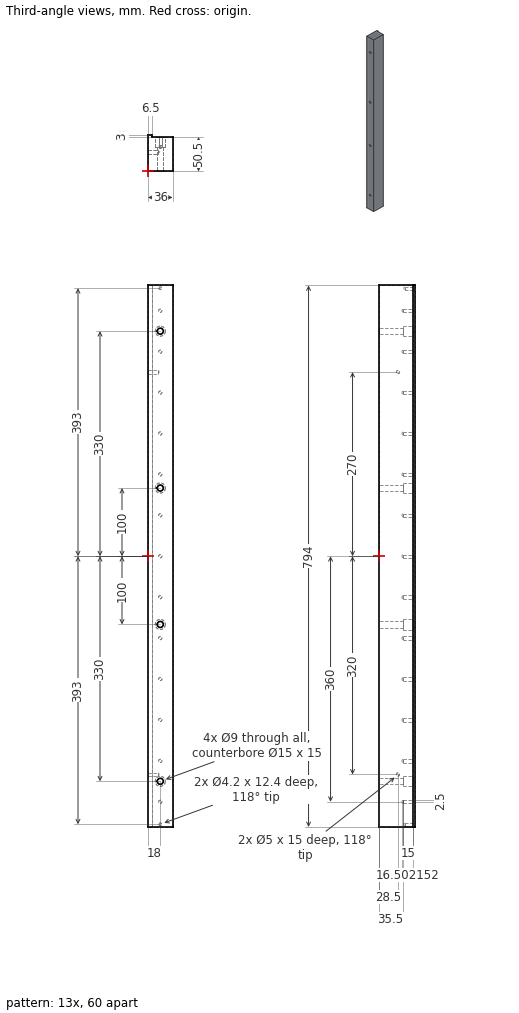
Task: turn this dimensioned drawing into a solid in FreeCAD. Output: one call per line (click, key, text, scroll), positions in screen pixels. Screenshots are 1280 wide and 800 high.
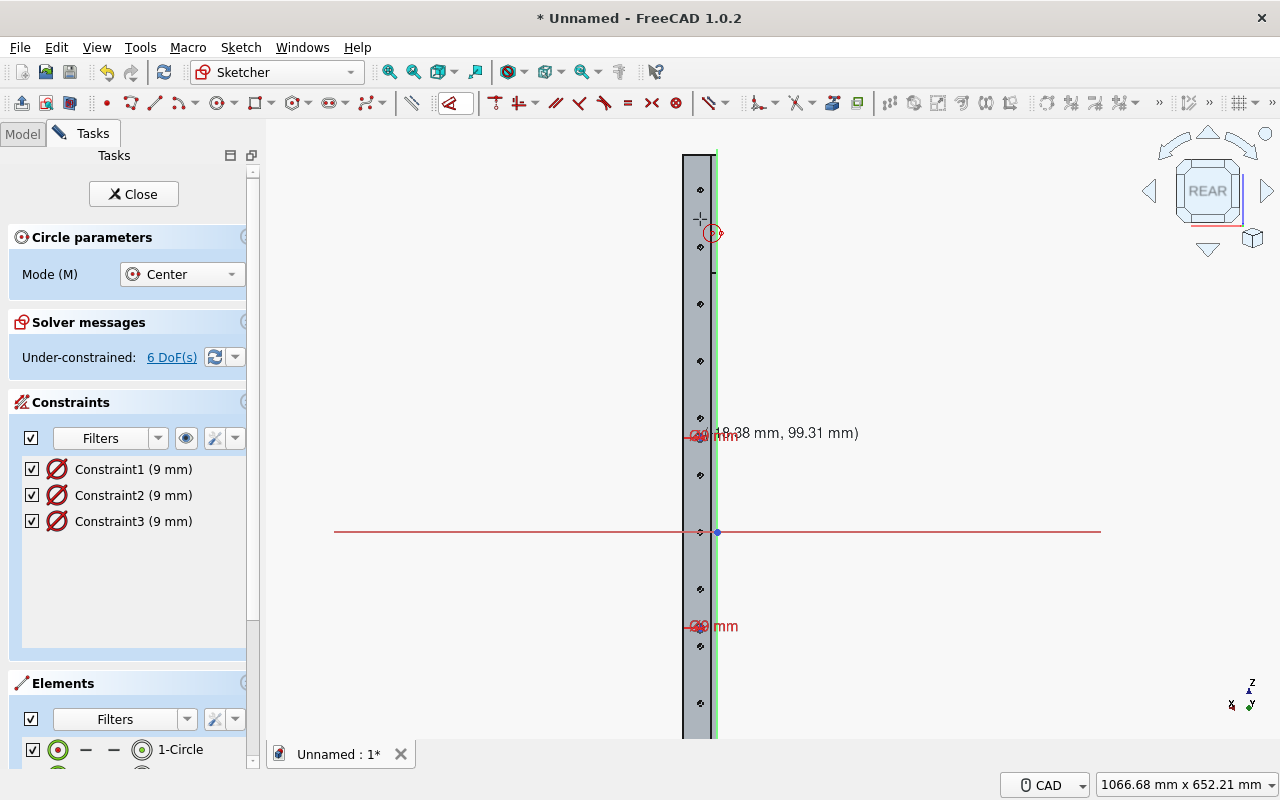
click(700, 219)
move(703, 216)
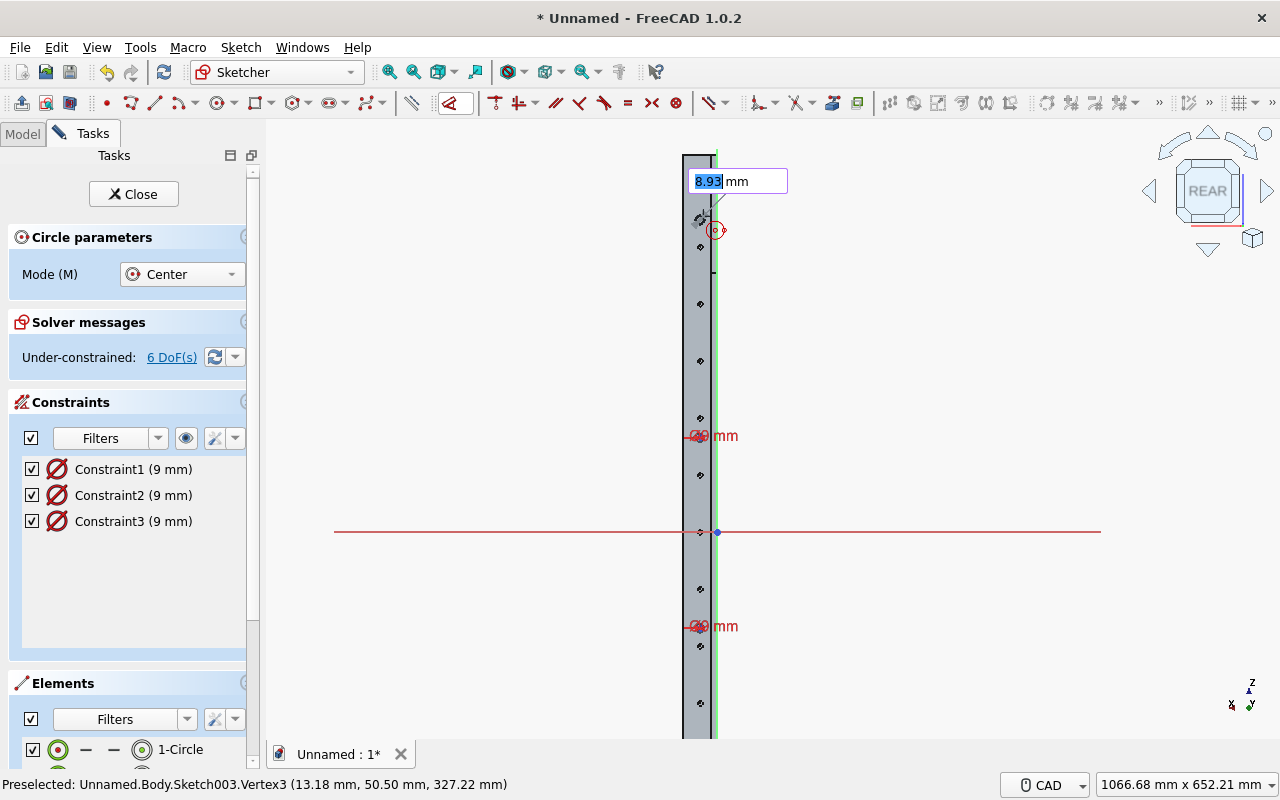
text(9)
key(Return)
key(Escape)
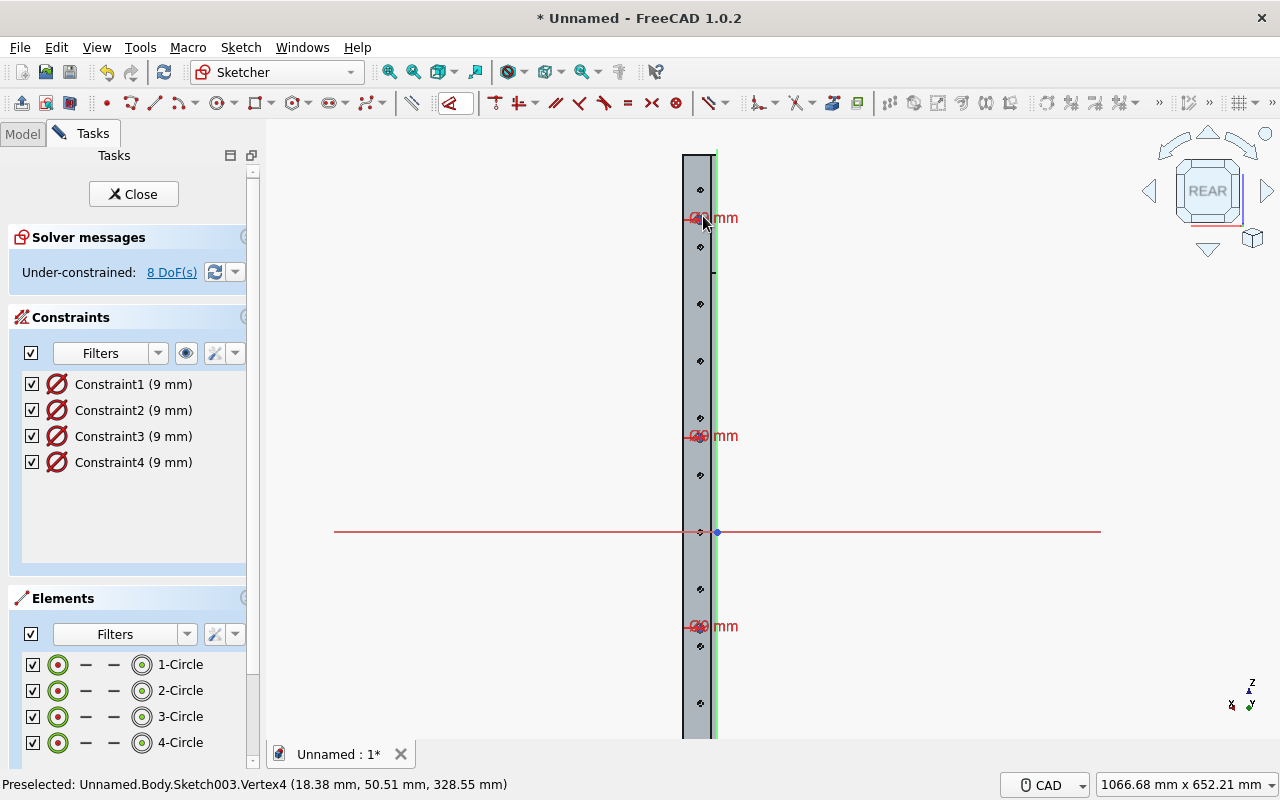
scroll(700, 219, down, 2)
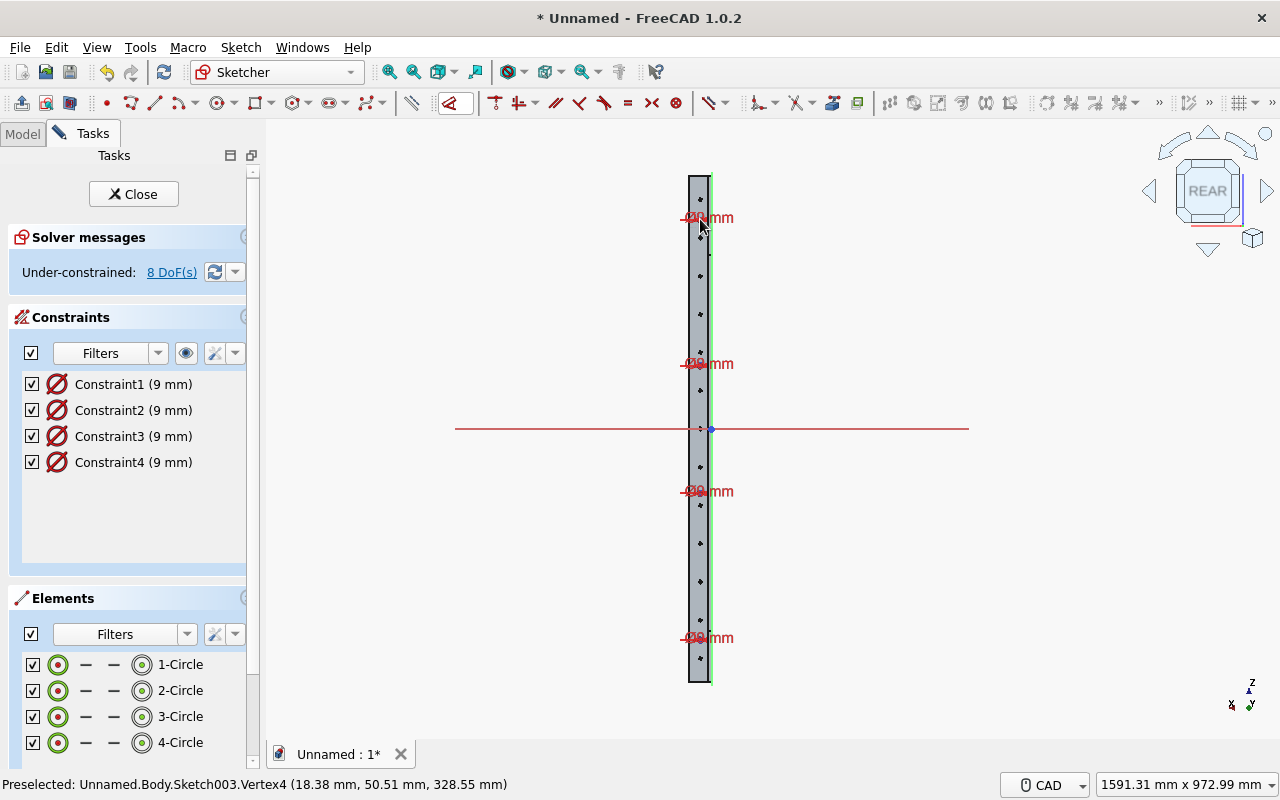
click(700, 640)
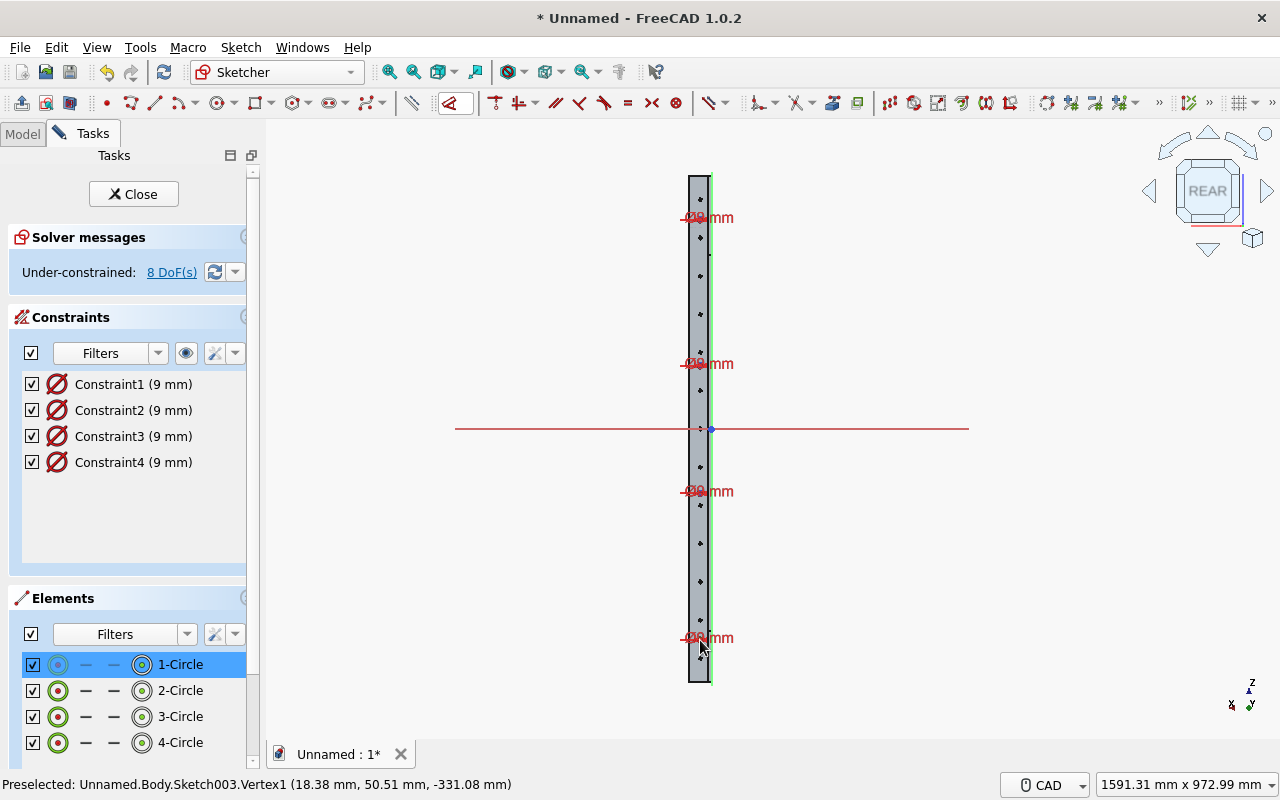
click(700, 493)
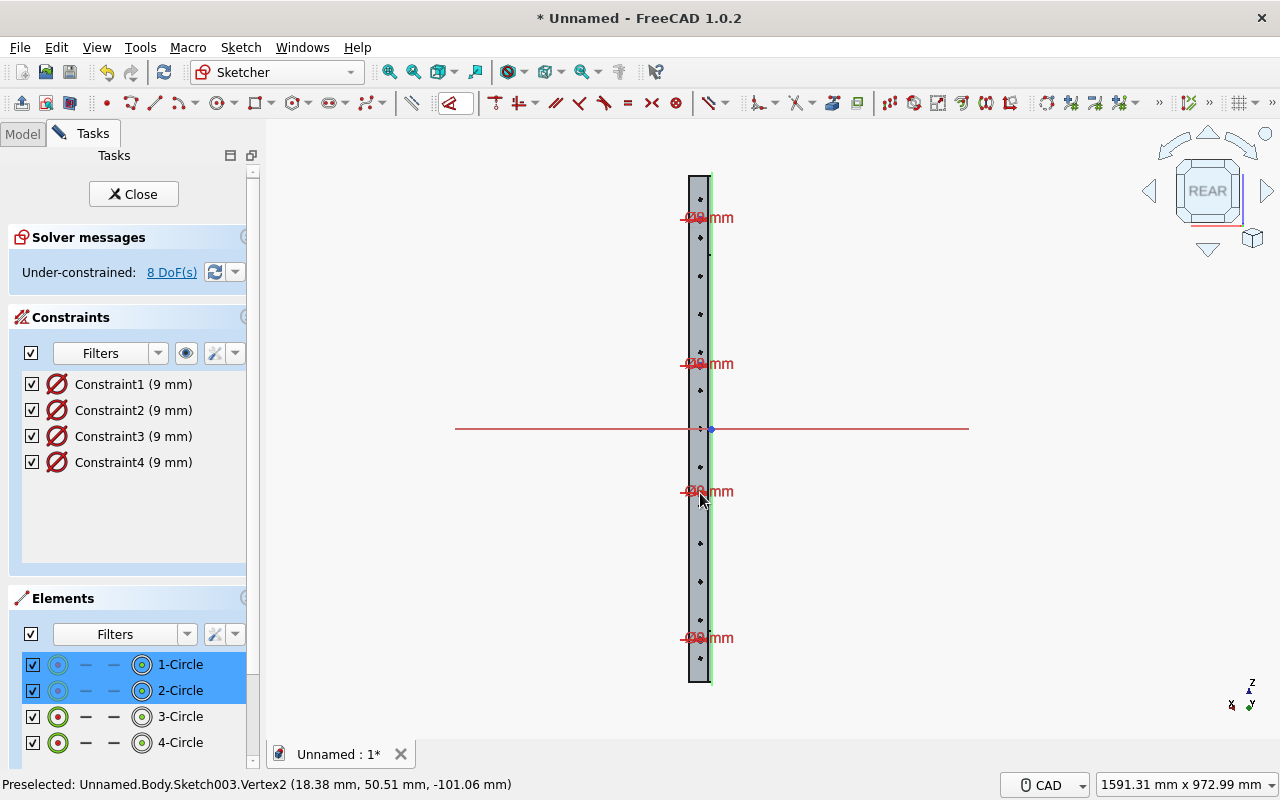
click(538, 104)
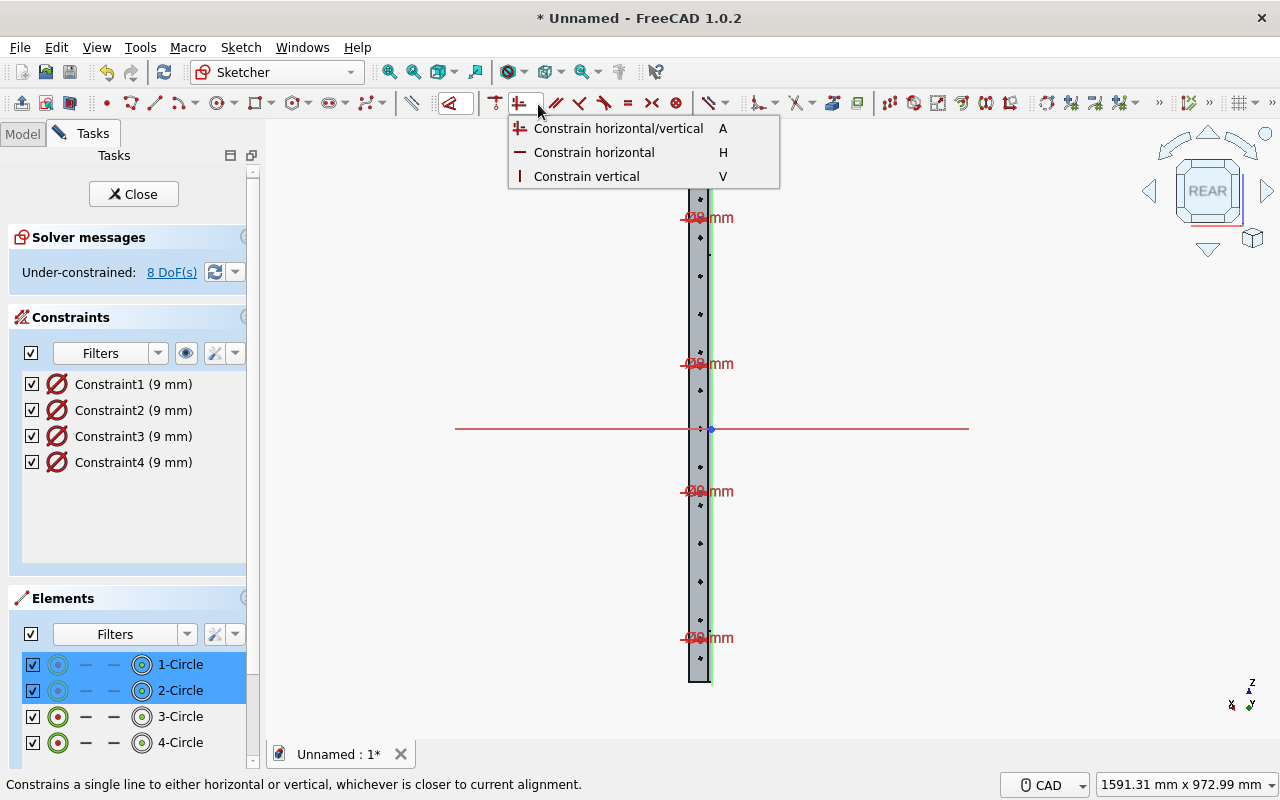
click(644, 176)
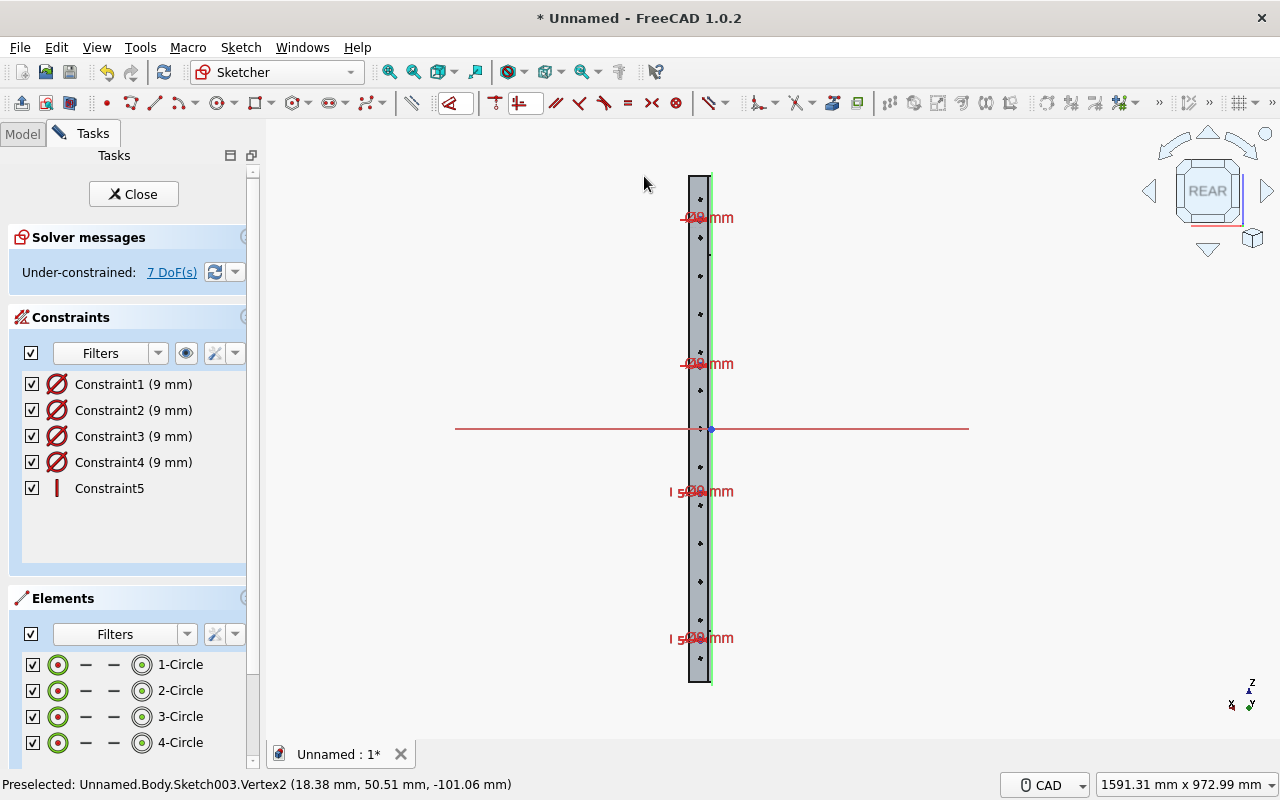
click(700, 493)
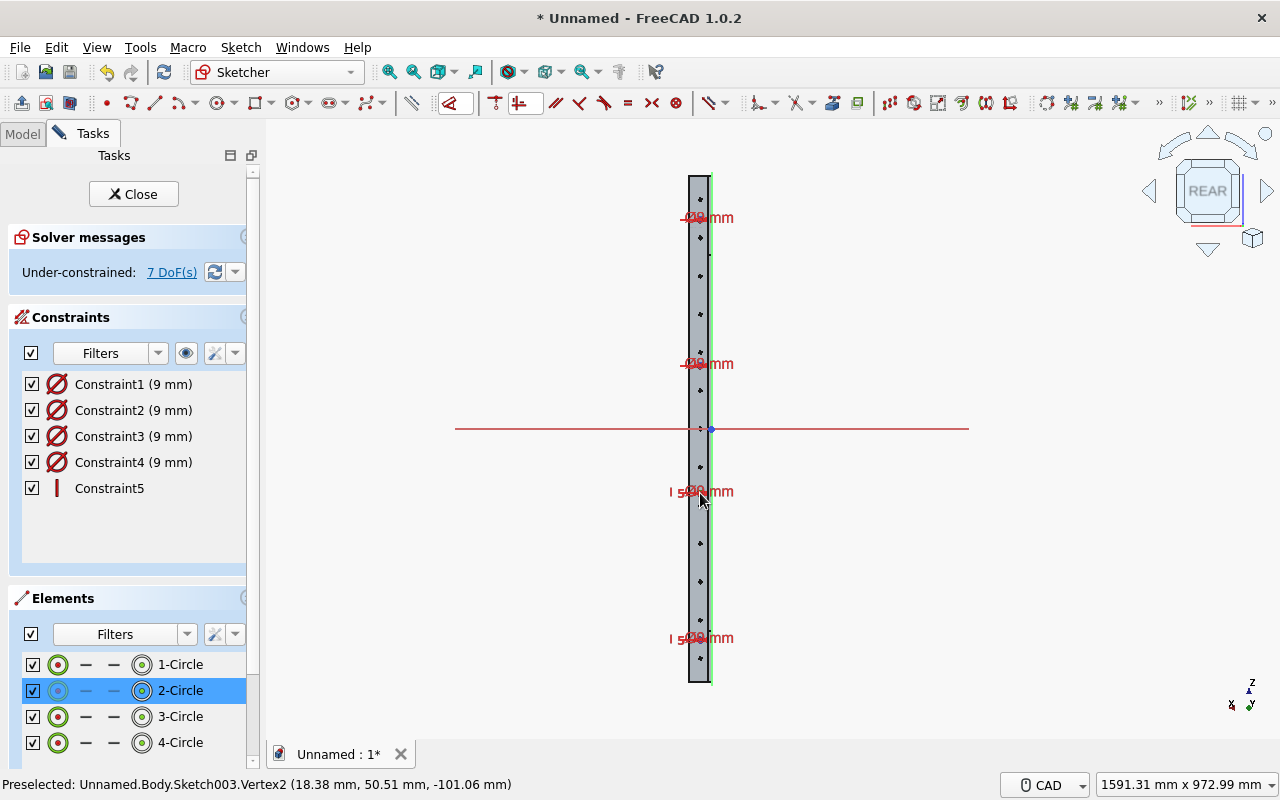
click(700, 366)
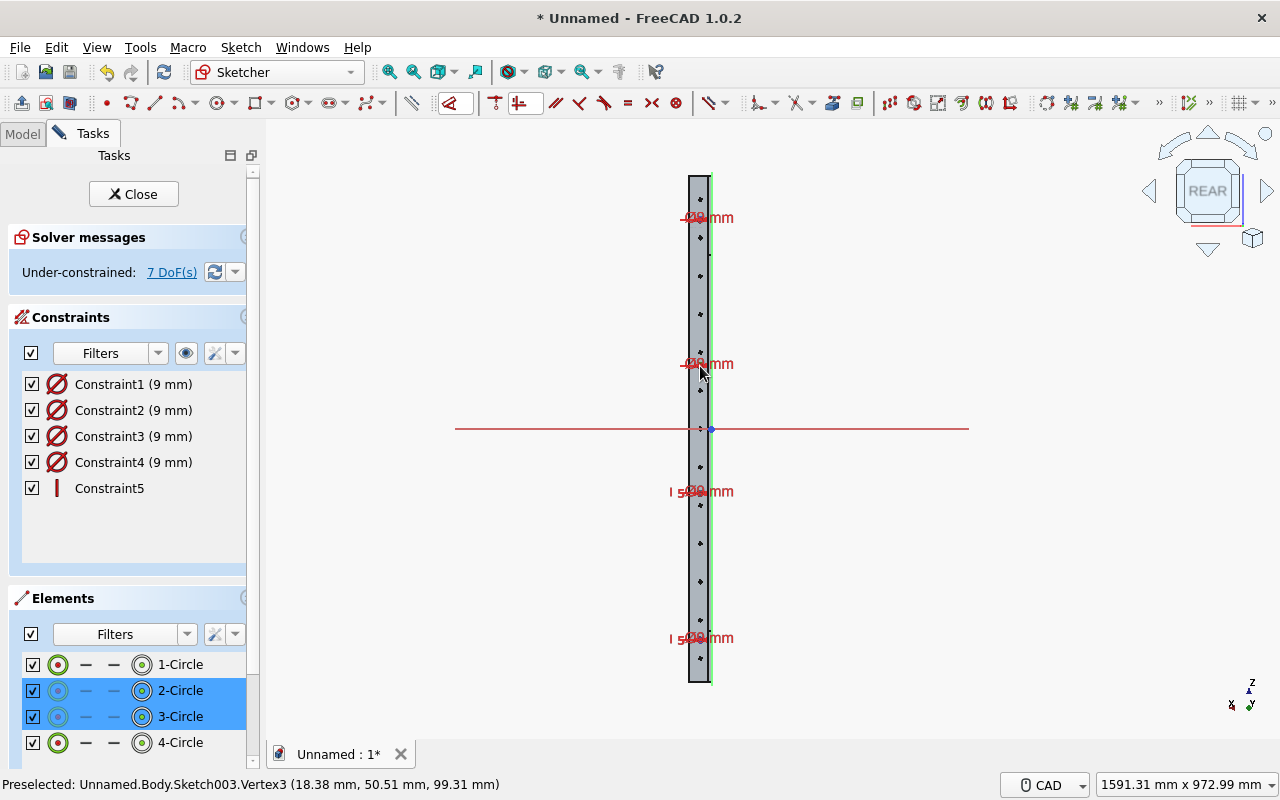
key(v)